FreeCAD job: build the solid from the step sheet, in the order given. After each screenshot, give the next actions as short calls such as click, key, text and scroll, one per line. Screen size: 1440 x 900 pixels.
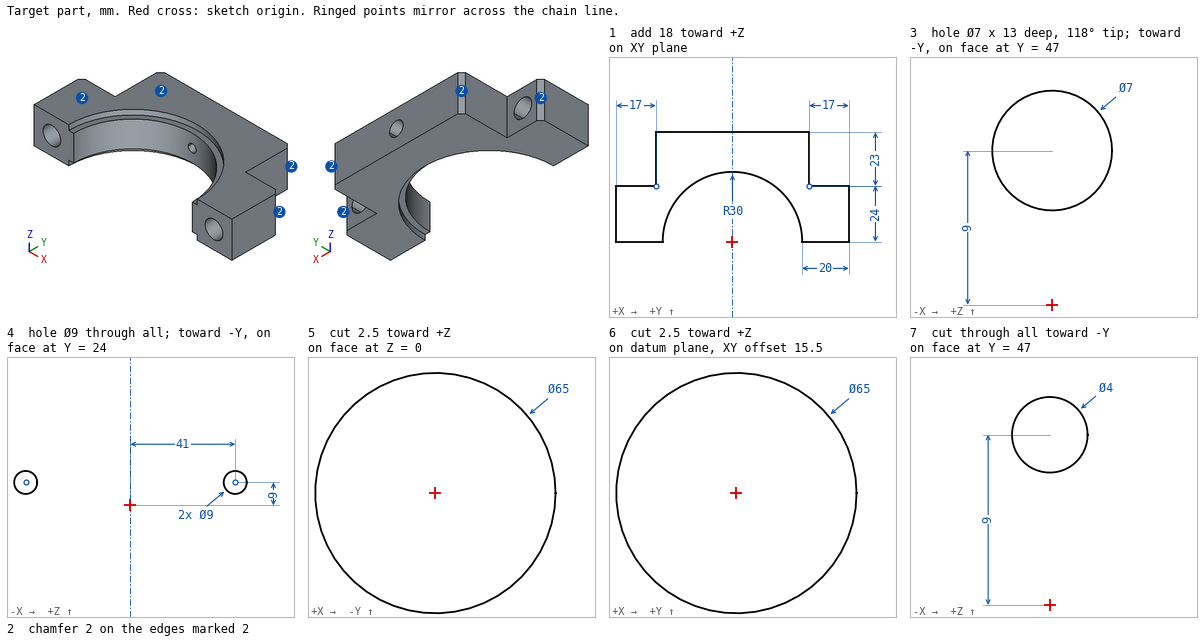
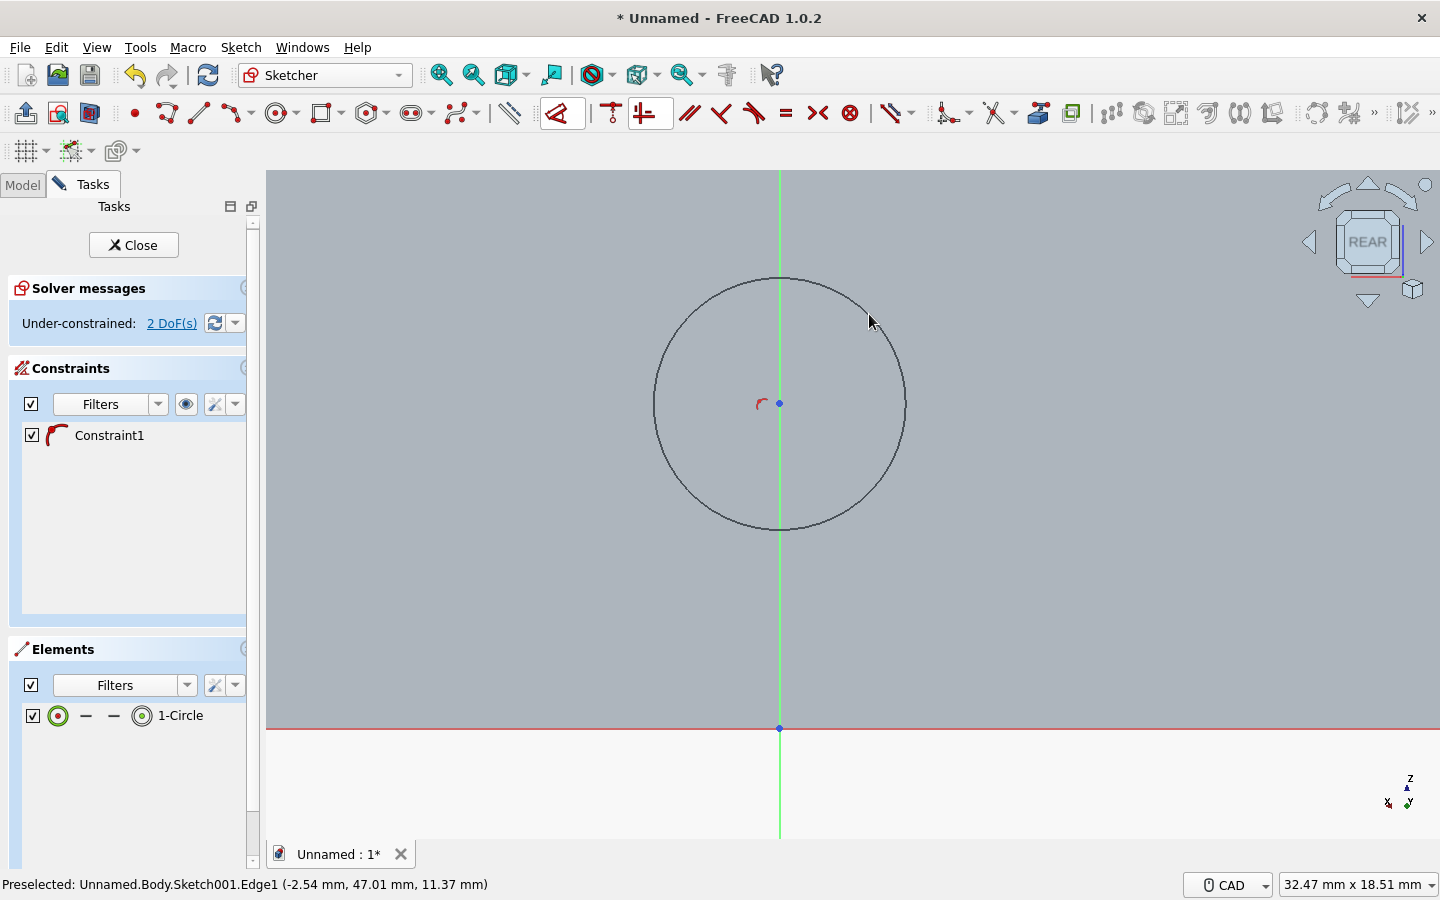
click(869, 315)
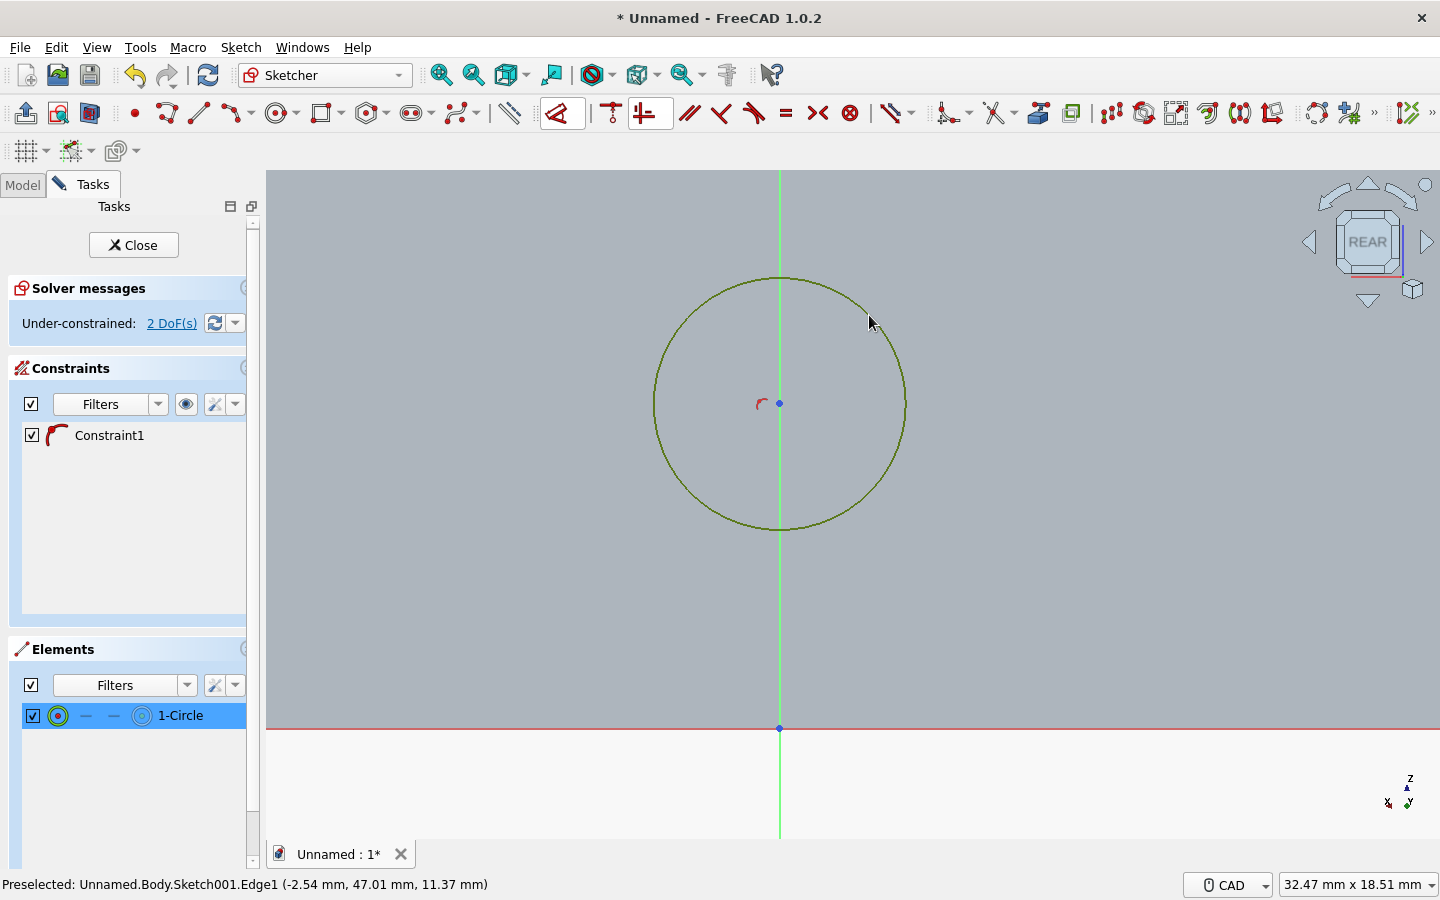
key(k)
key(o)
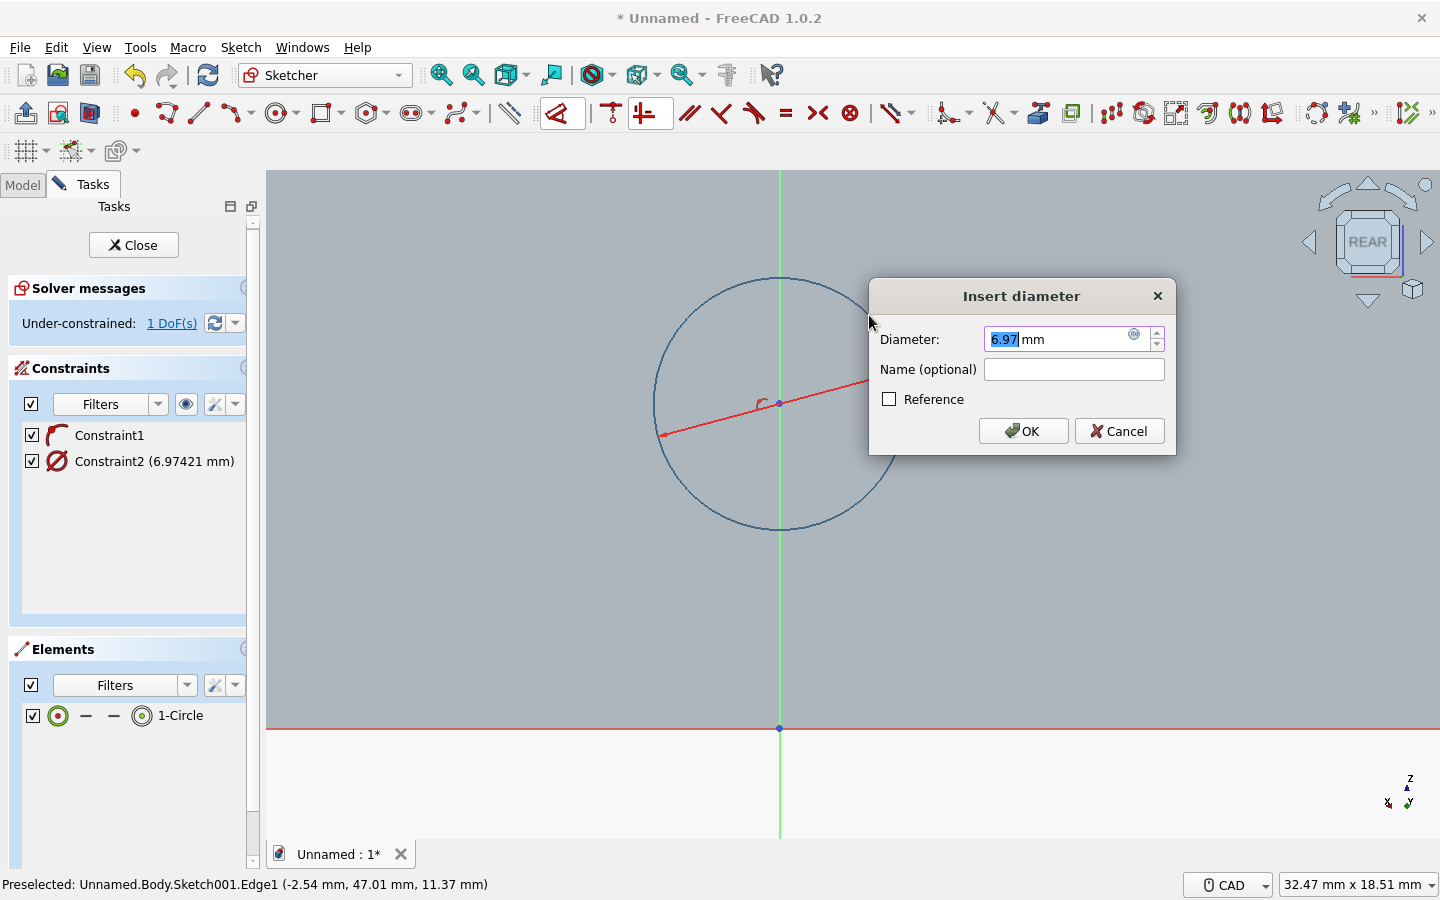
text(7)
key(Return)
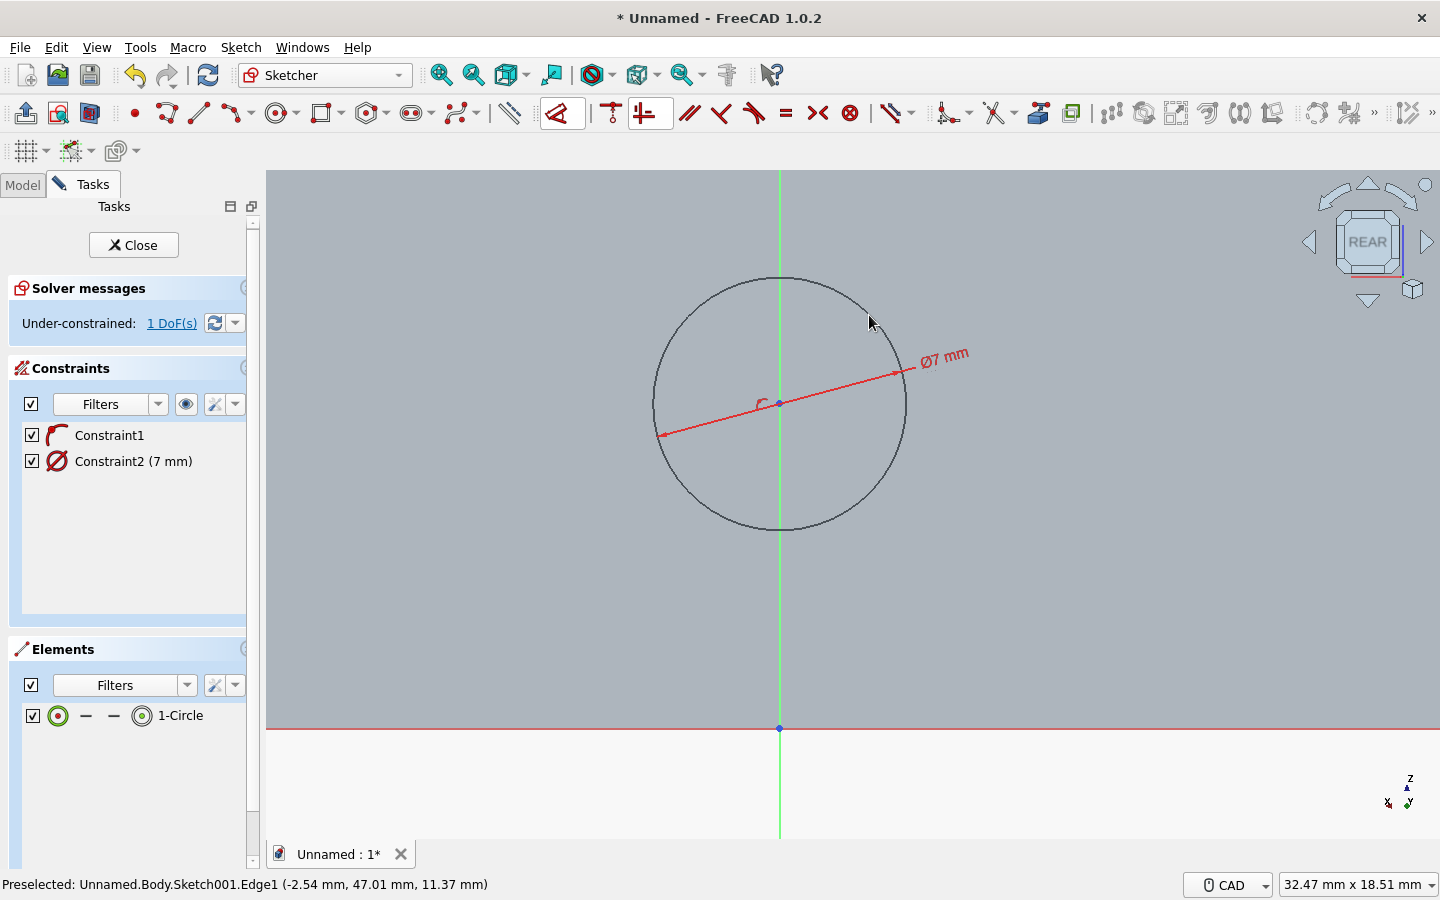
click(780, 404)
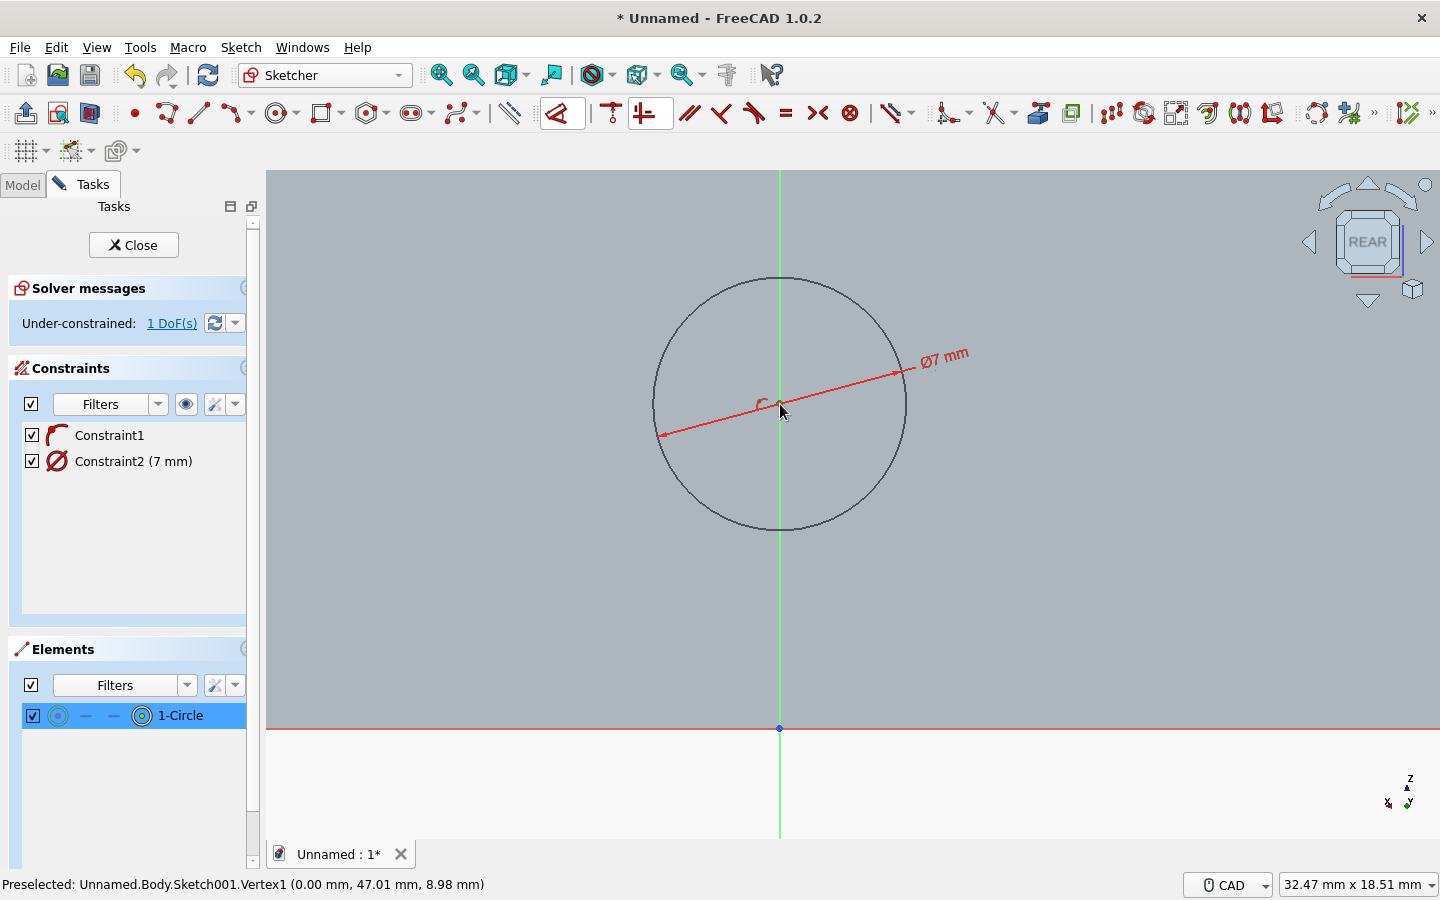
key(i)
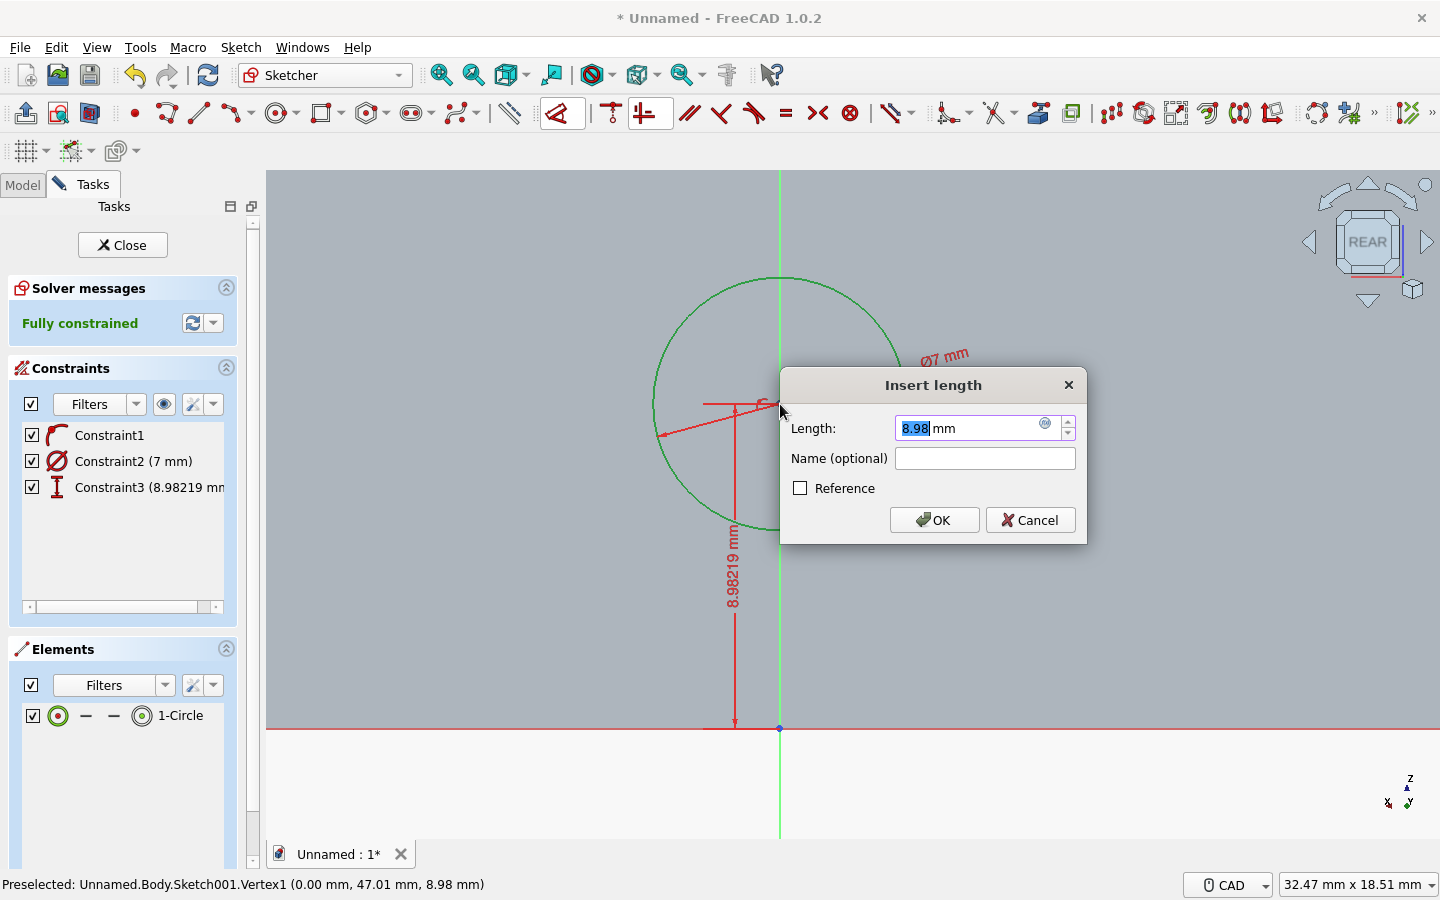
text(9)
key(Return)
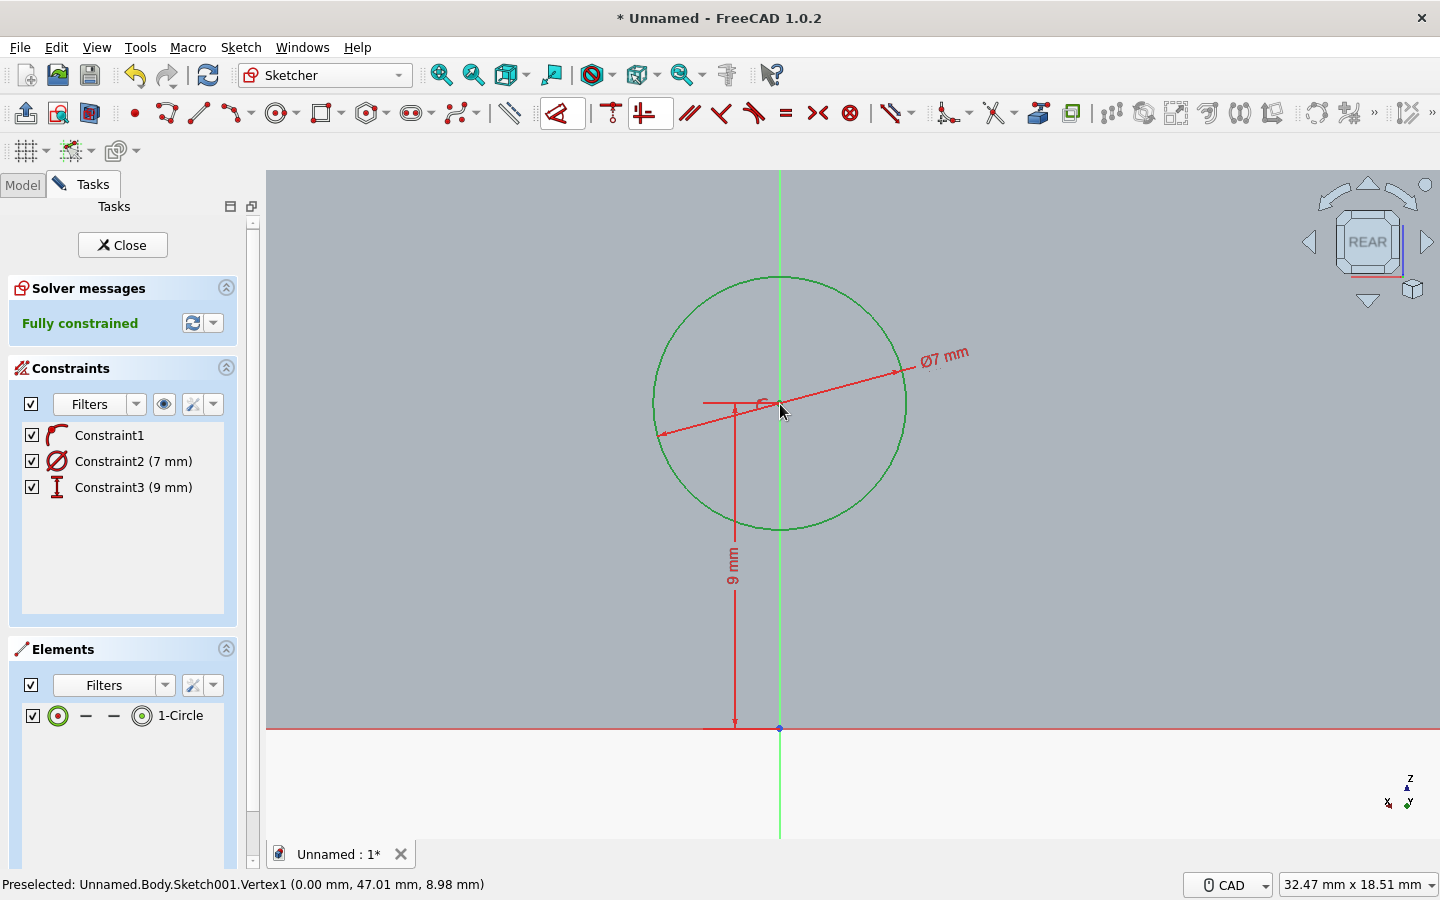
click(123, 245)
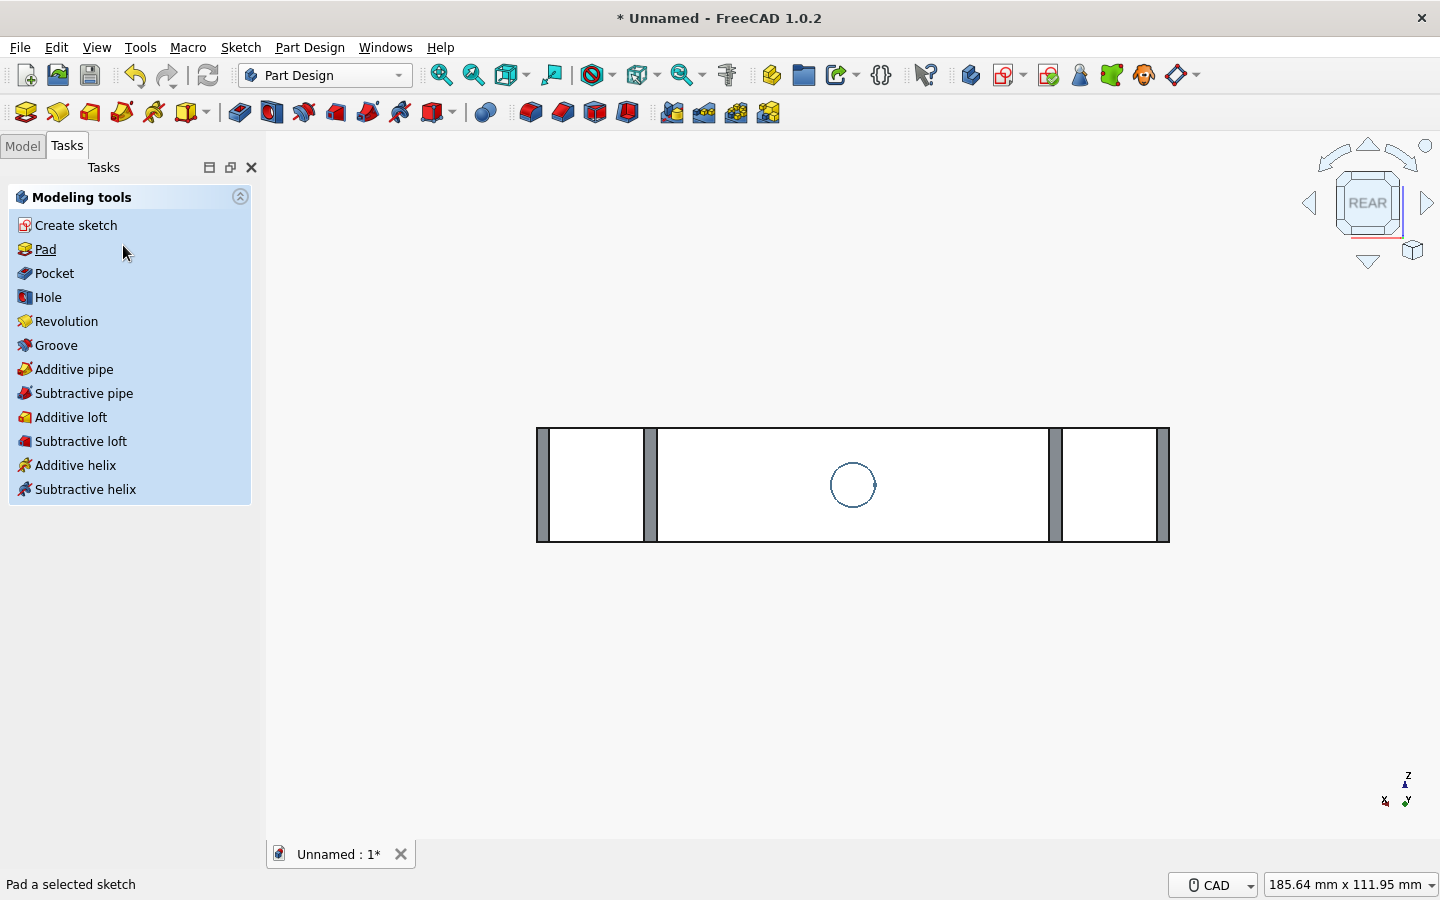
click(272, 112)